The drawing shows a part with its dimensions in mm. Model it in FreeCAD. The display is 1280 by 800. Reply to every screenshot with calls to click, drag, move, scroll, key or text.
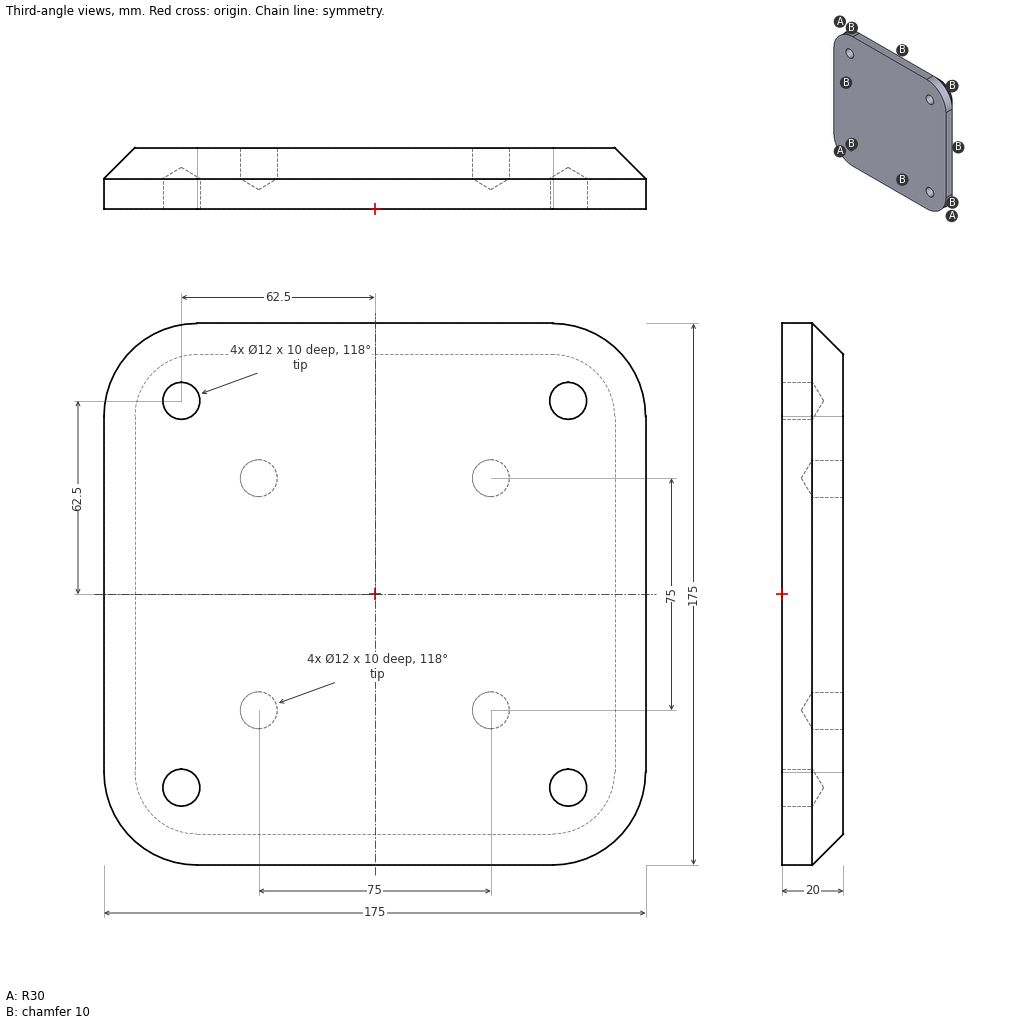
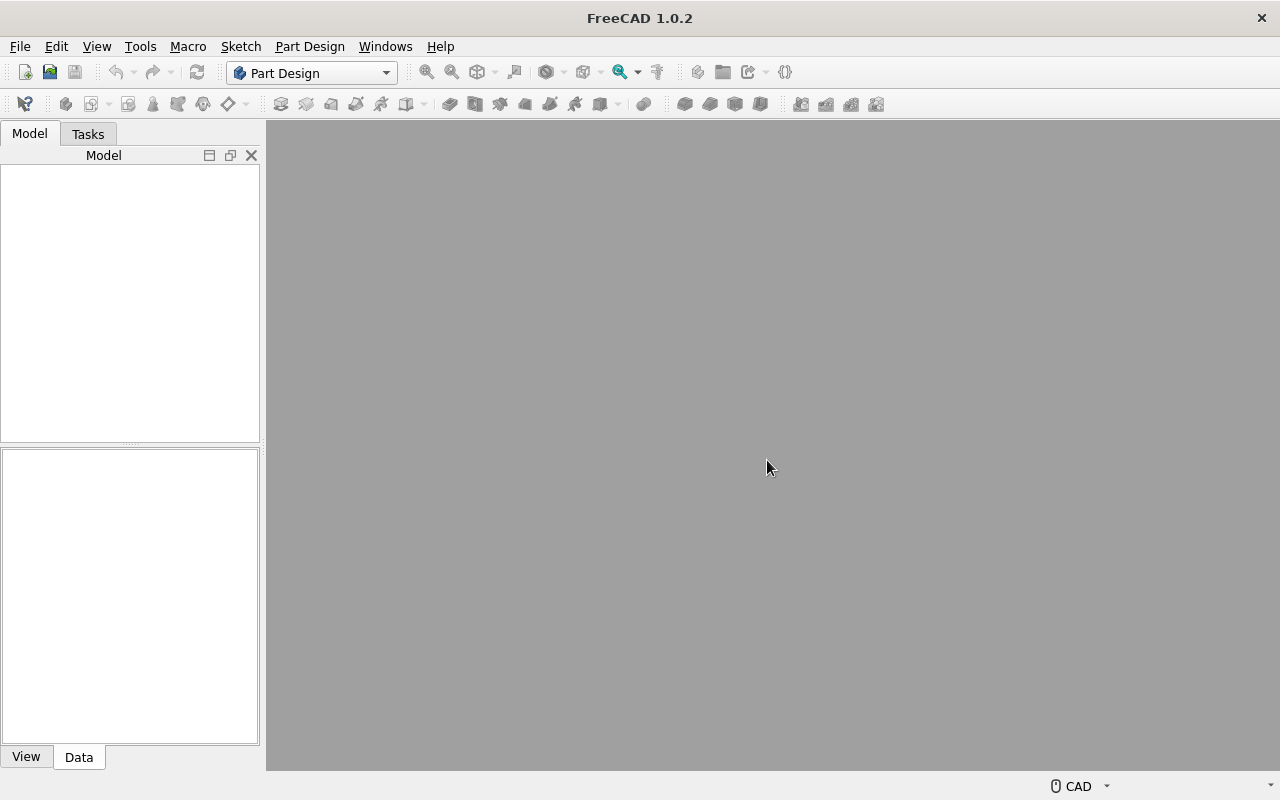
click(25, 72)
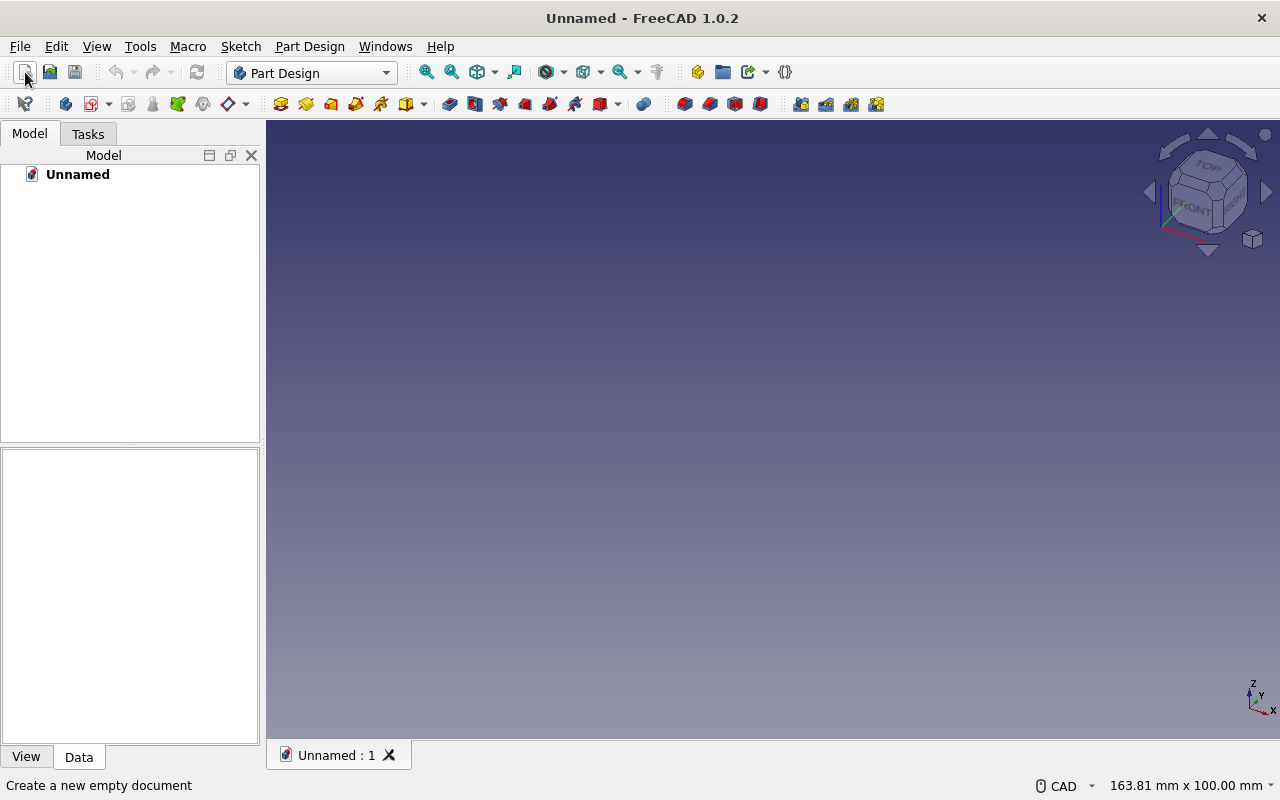
click(90, 104)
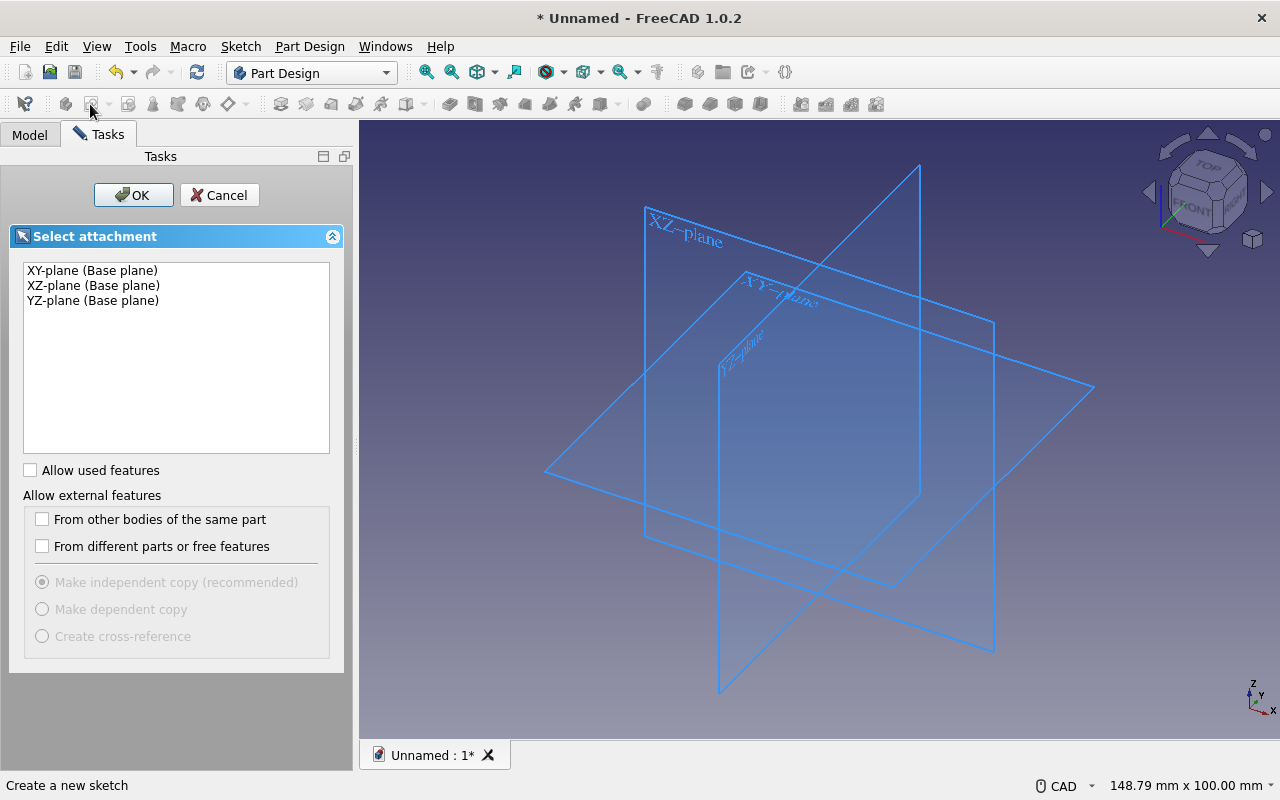
click(84, 286)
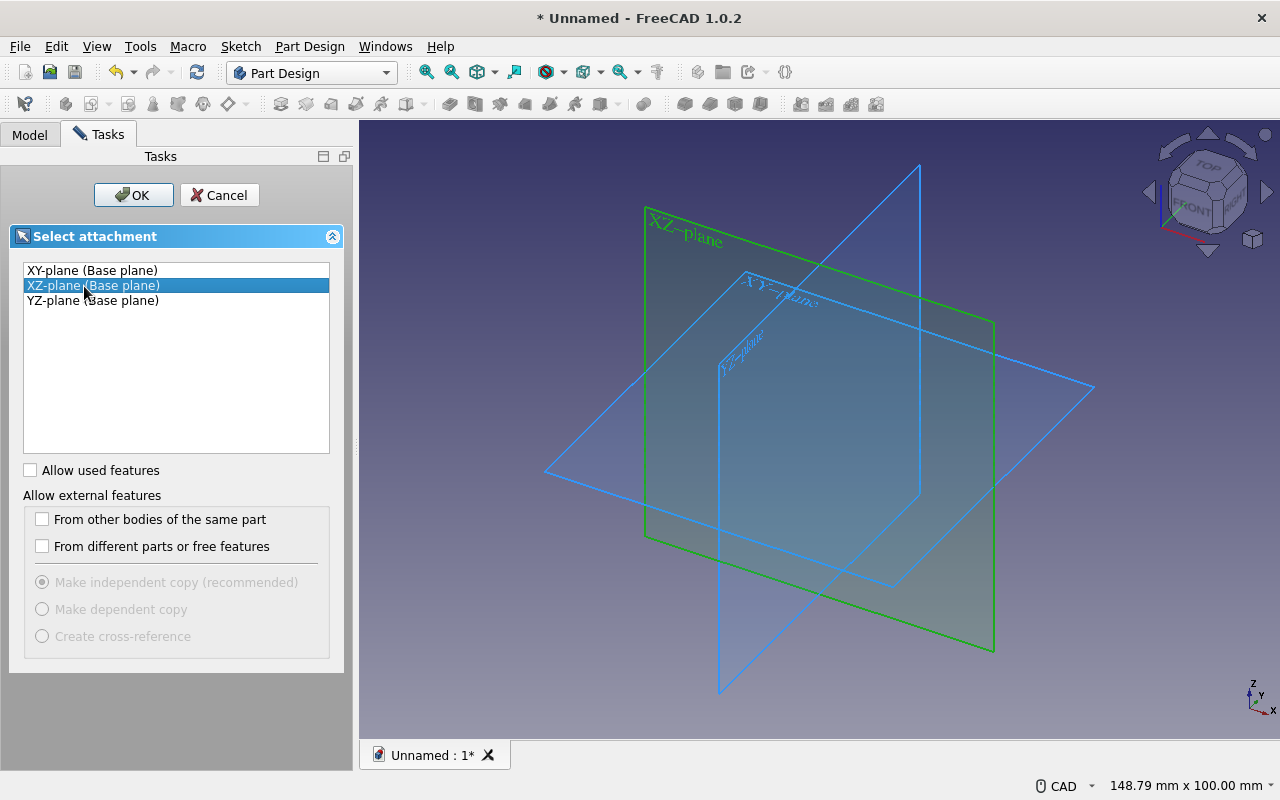
click(134, 195)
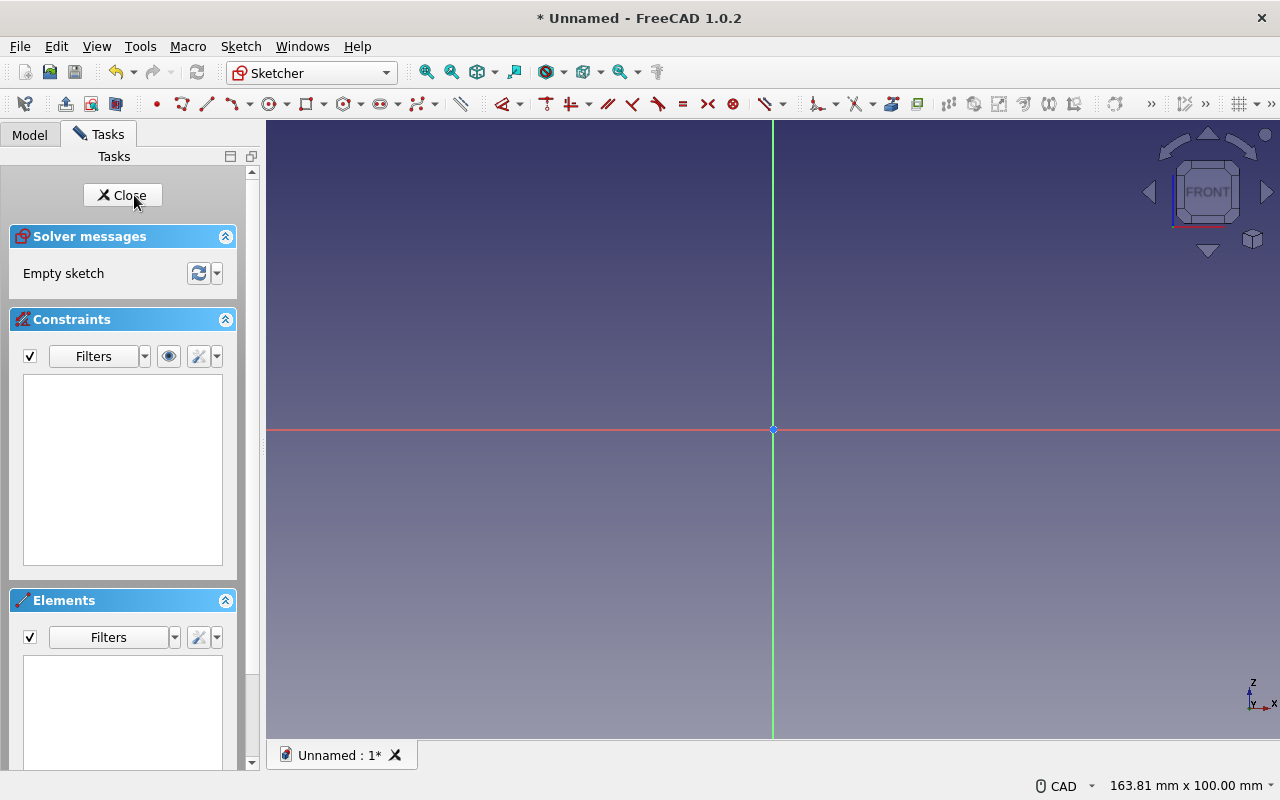
scroll(665, 430, down, 5)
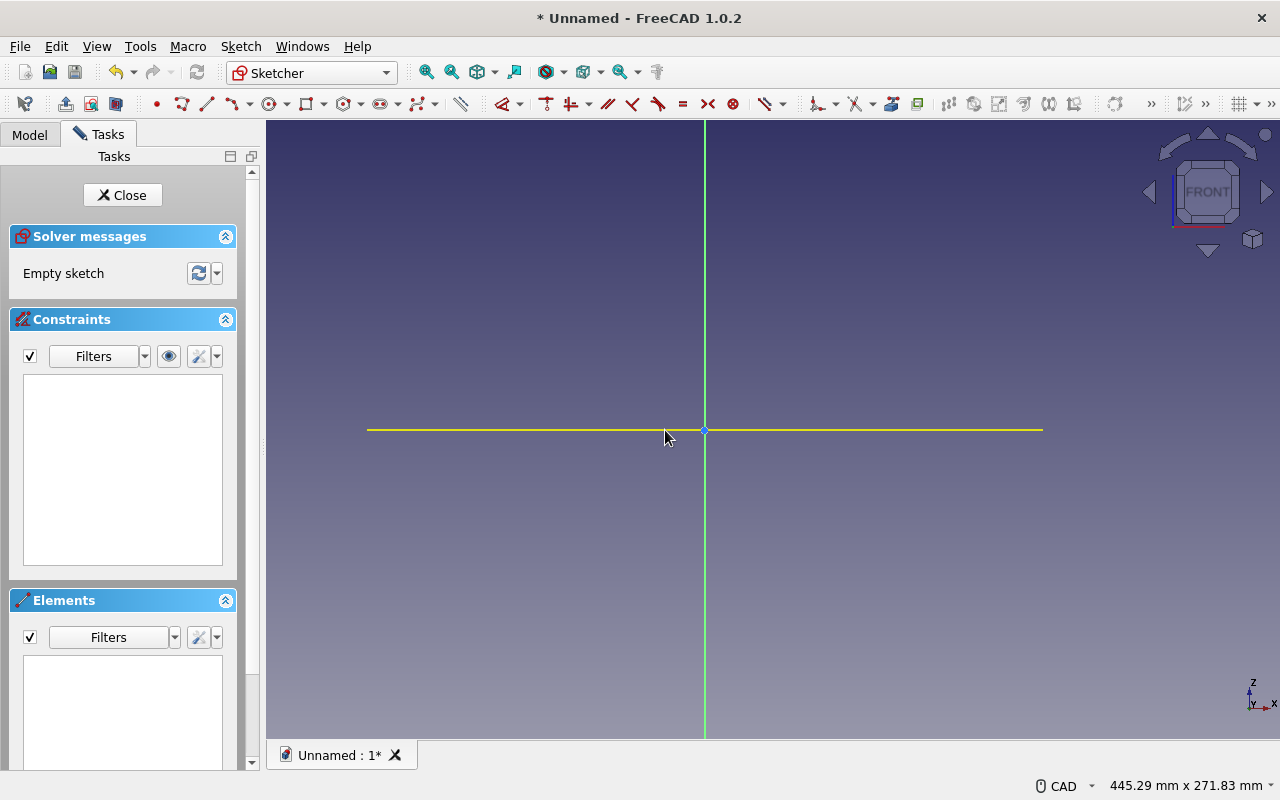
click(324, 104)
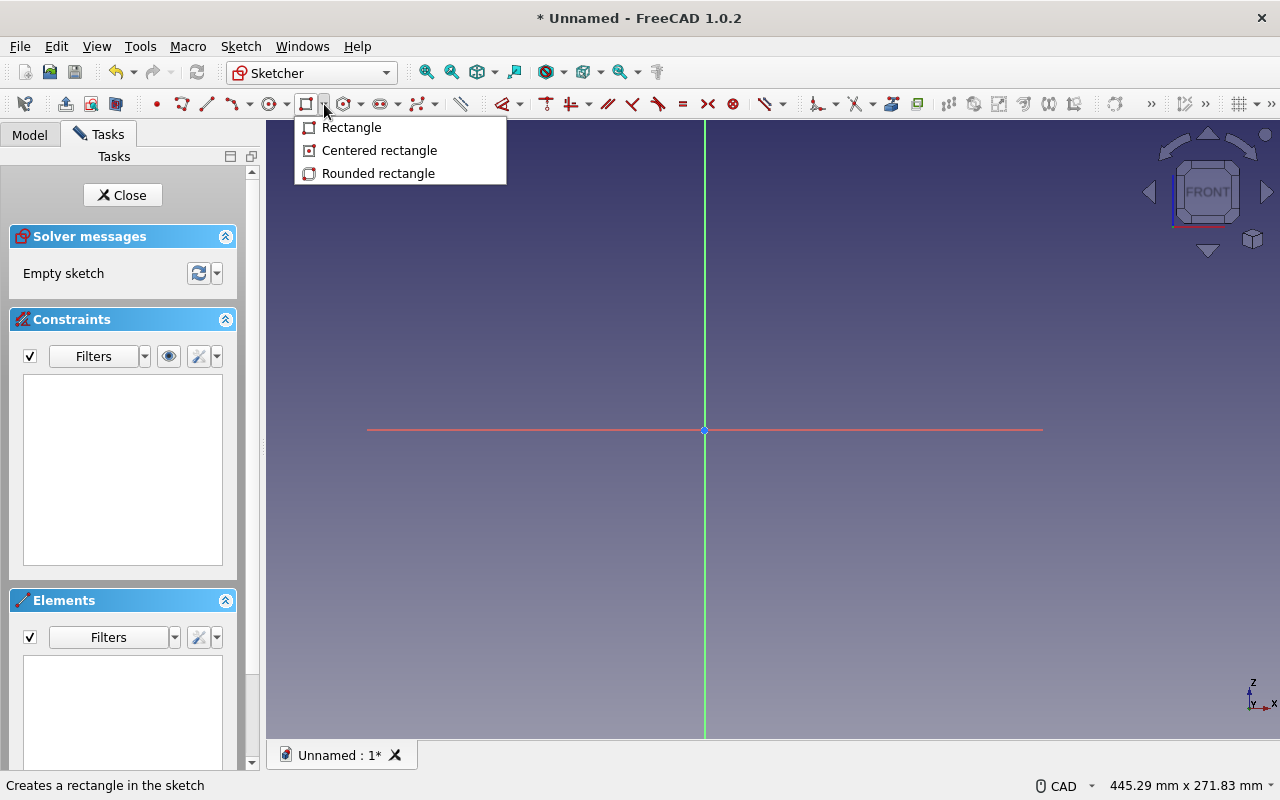
click(400, 150)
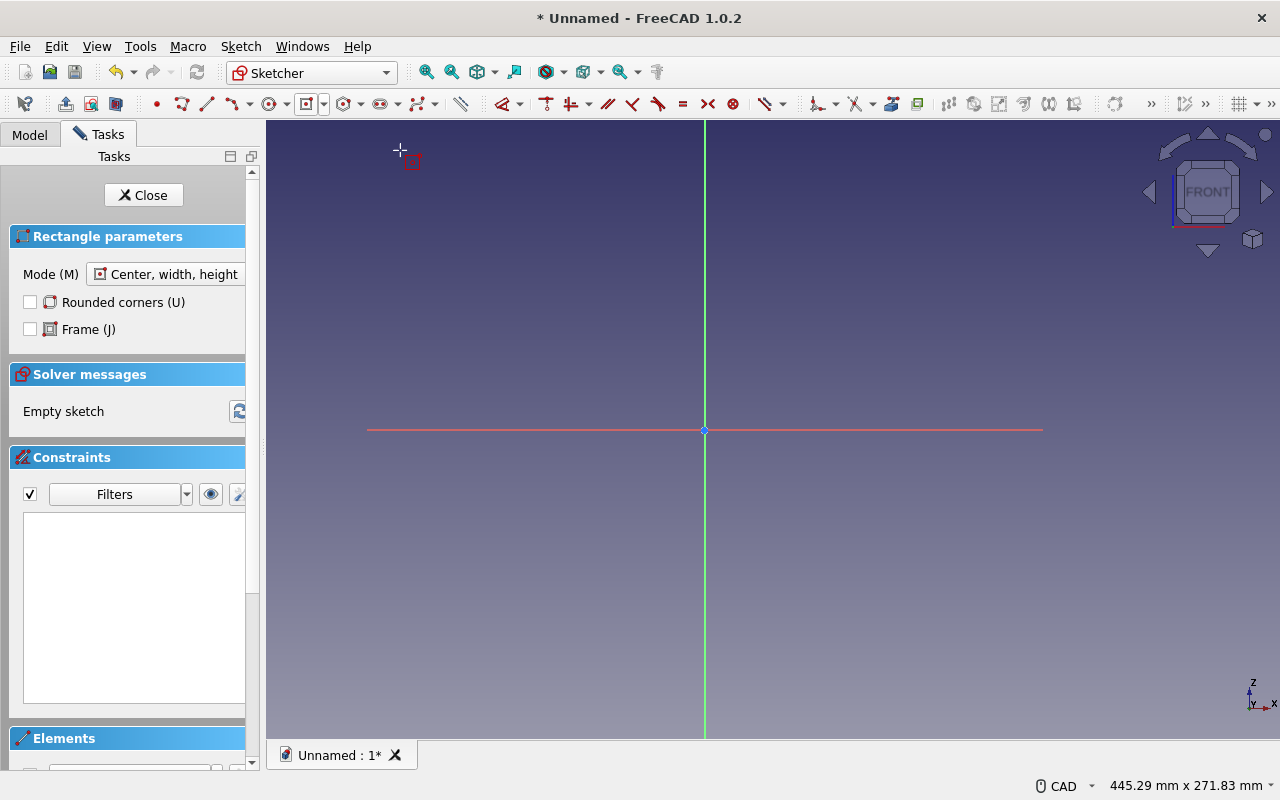
click(705, 430)
click(904, 231)
key(Escape)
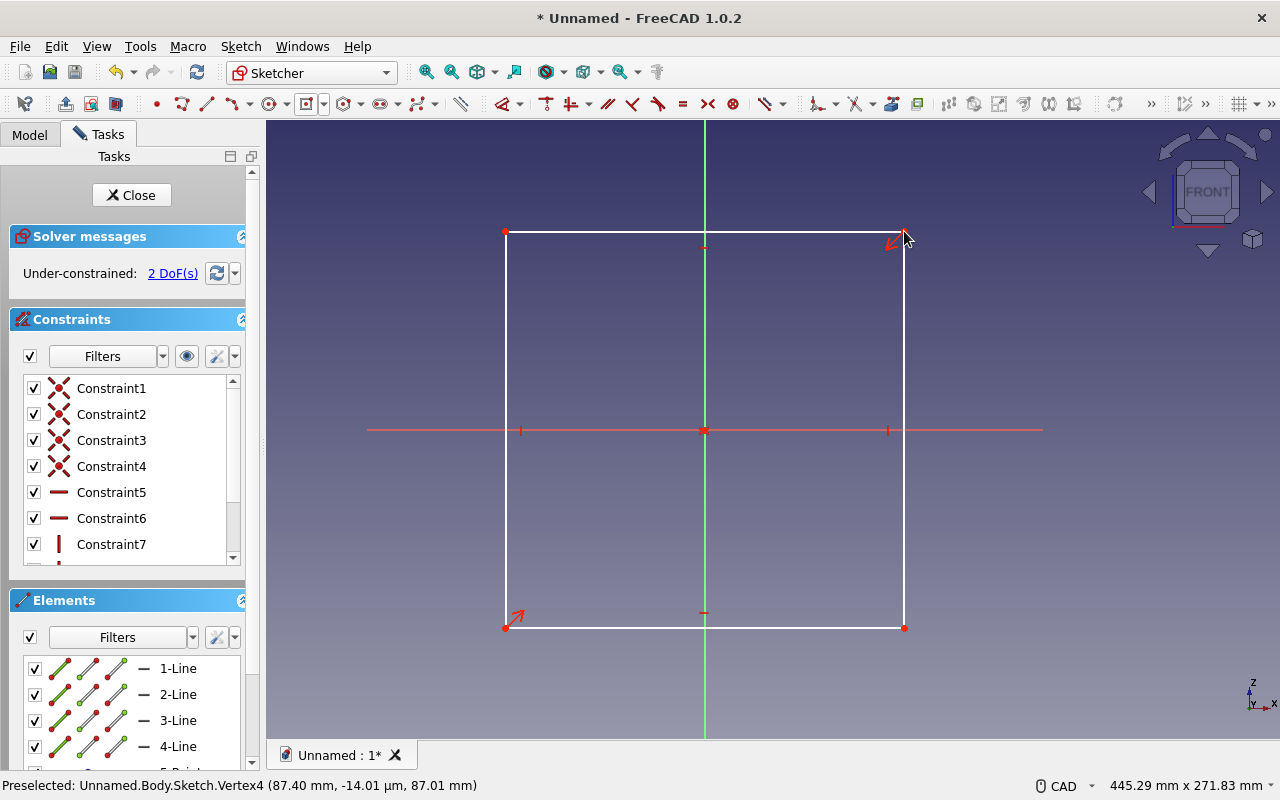
click(625, 628)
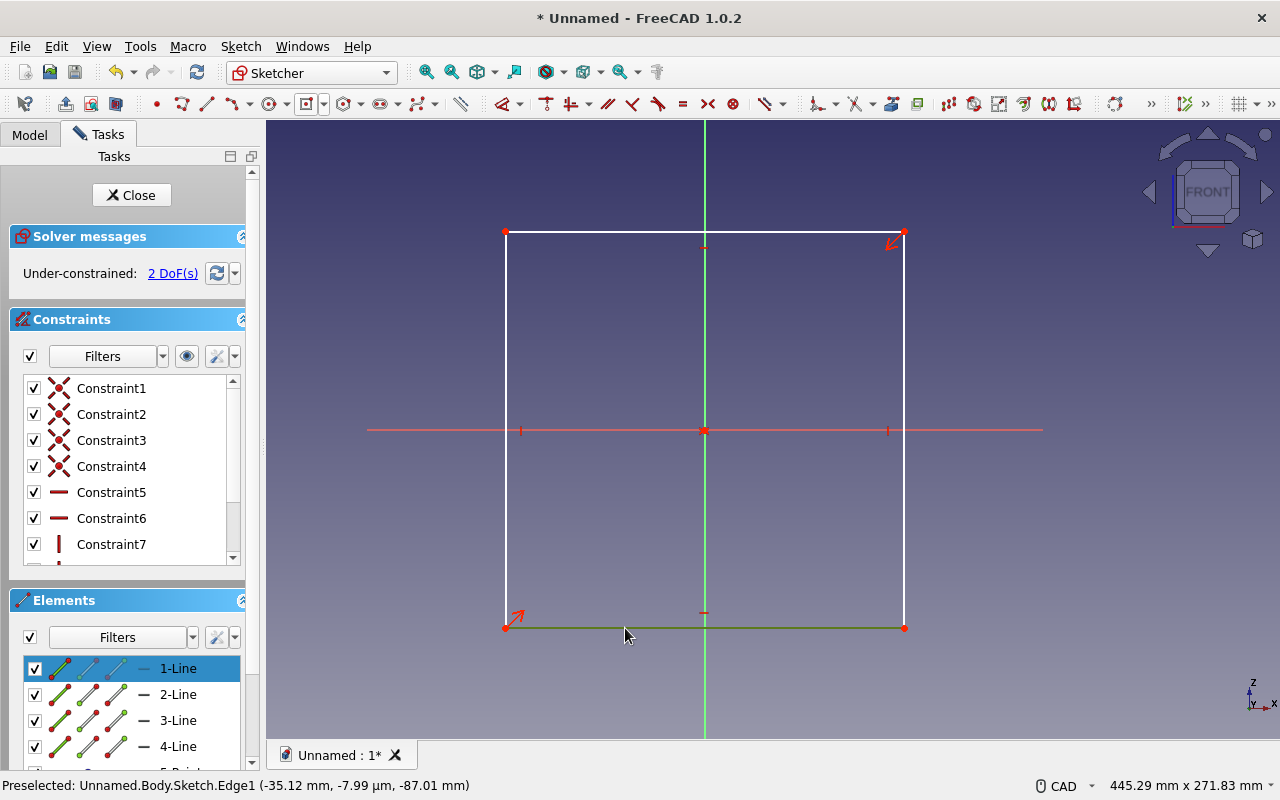
click(520, 104)